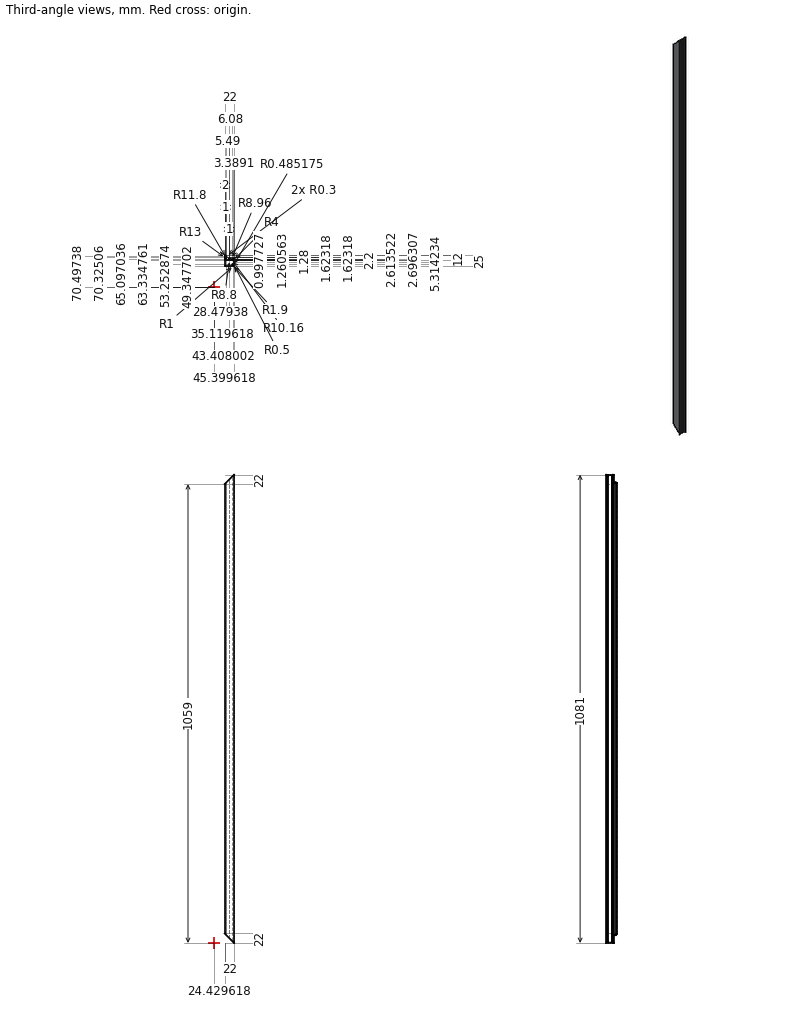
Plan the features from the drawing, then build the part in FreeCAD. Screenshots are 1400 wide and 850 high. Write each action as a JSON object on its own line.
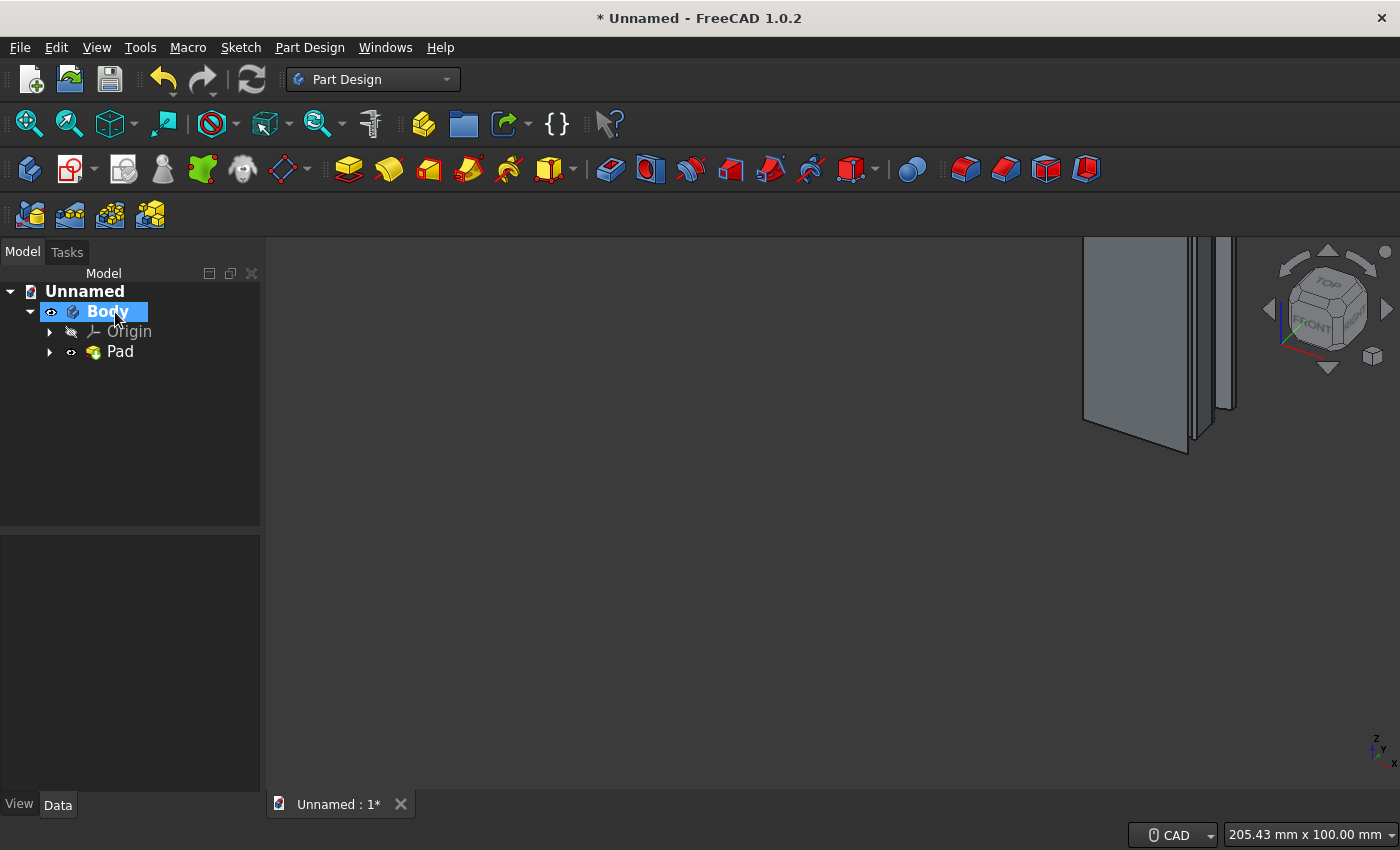
{"action": "left_click", "coordinate": [30, 124]}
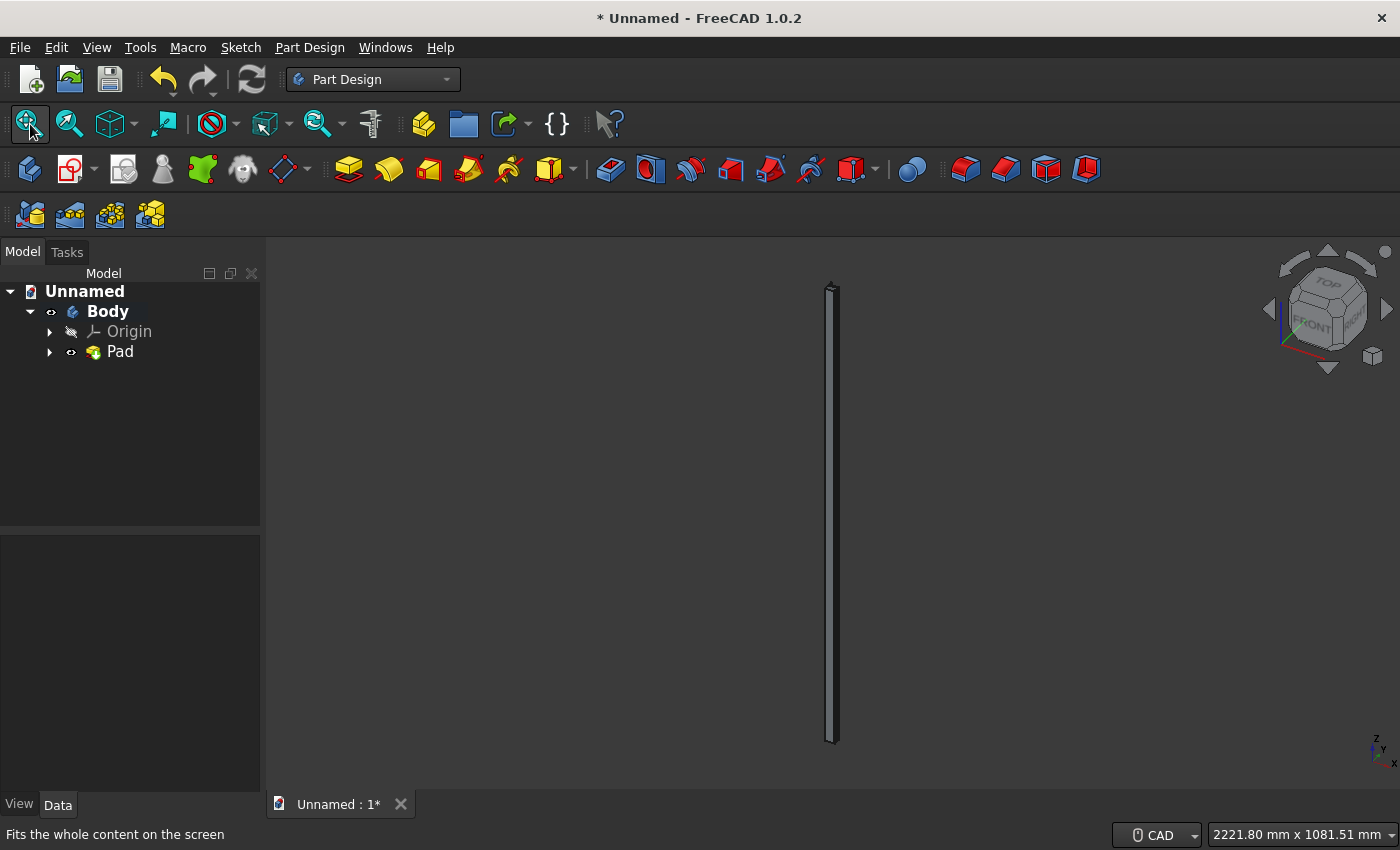
{"action": "scroll", "coordinate": [830, 321], "scroll_direction": "up", "scroll_amount": 4}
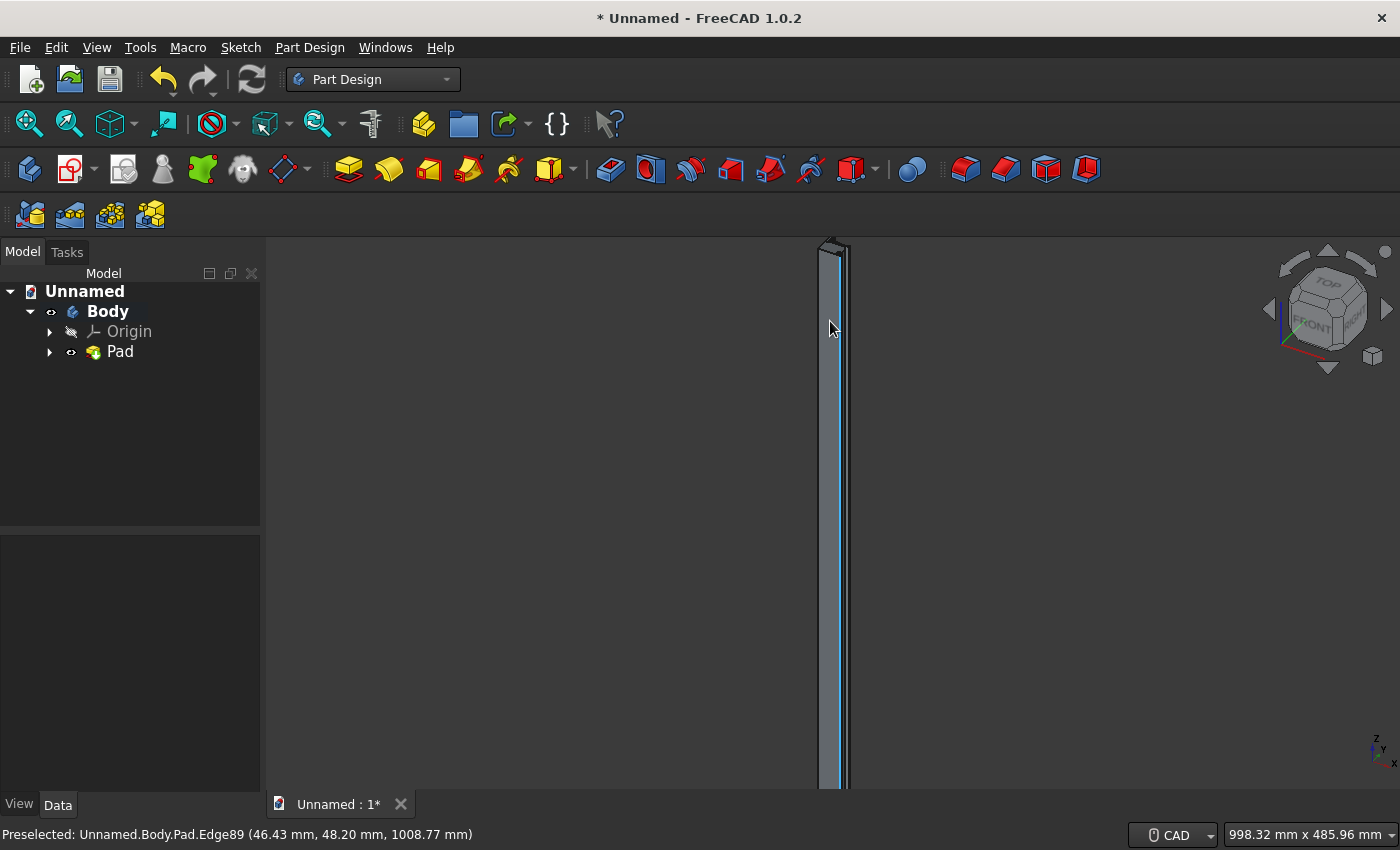
{"action": "left_click", "coordinate": [829, 323]}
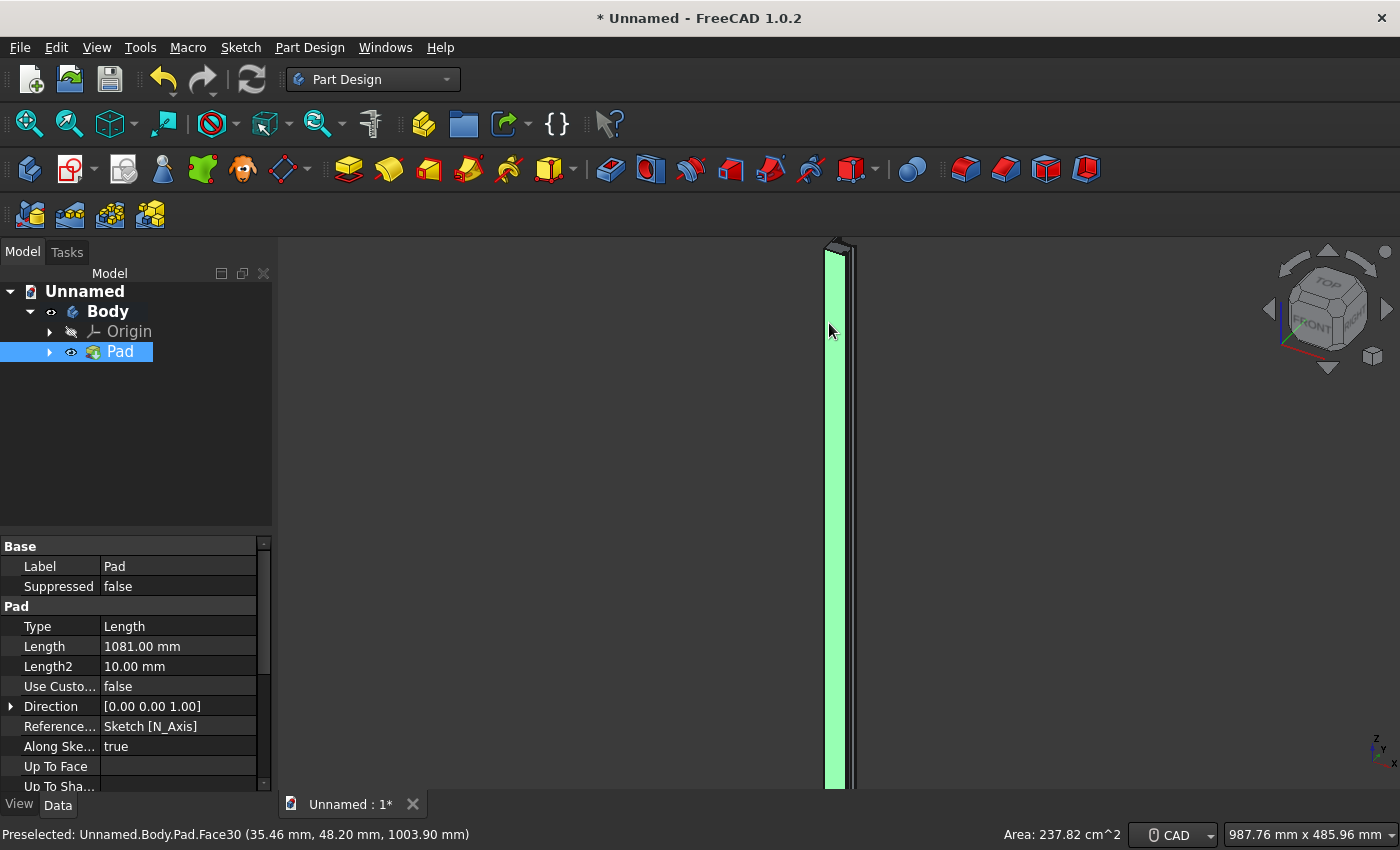
{"action": "left_click", "coordinate": [70, 170]}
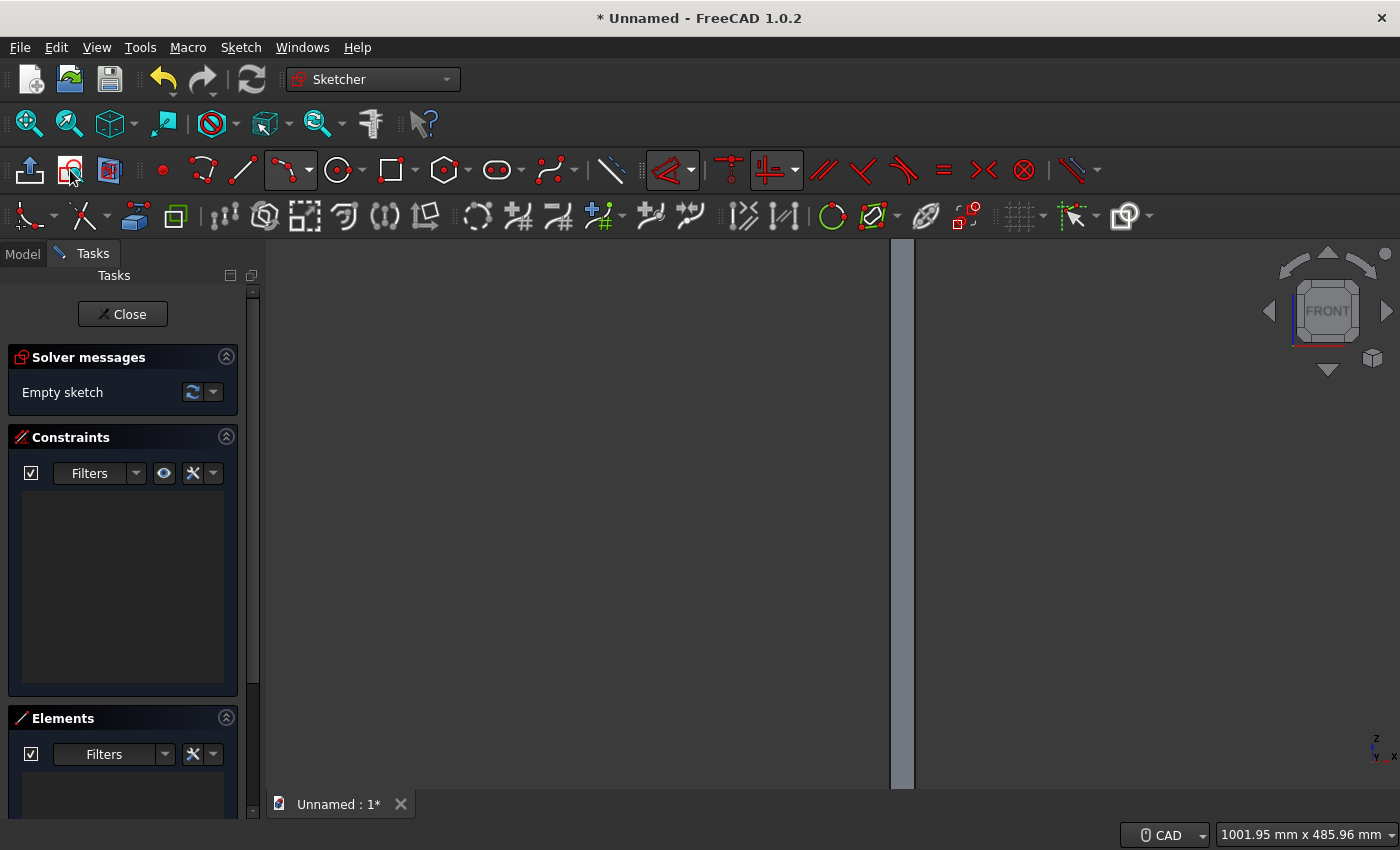
{"action": "scroll", "coordinate": [764, 514], "scroll_direction": "down", "scroll_amount": 5}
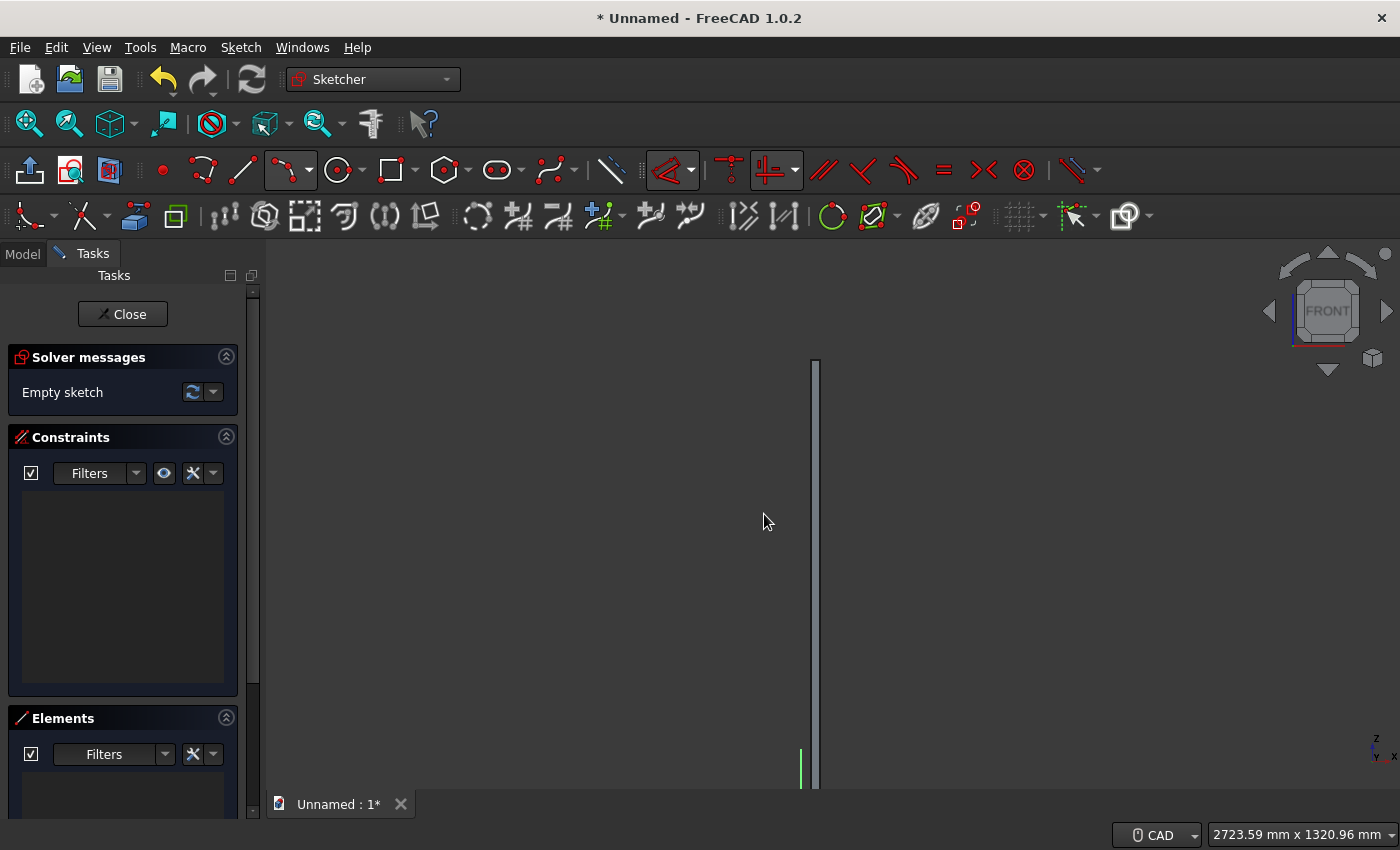
{"action": "scroll", "coordinate": [764, 514], "scroll_direction": "down", "scroll_amount": 5}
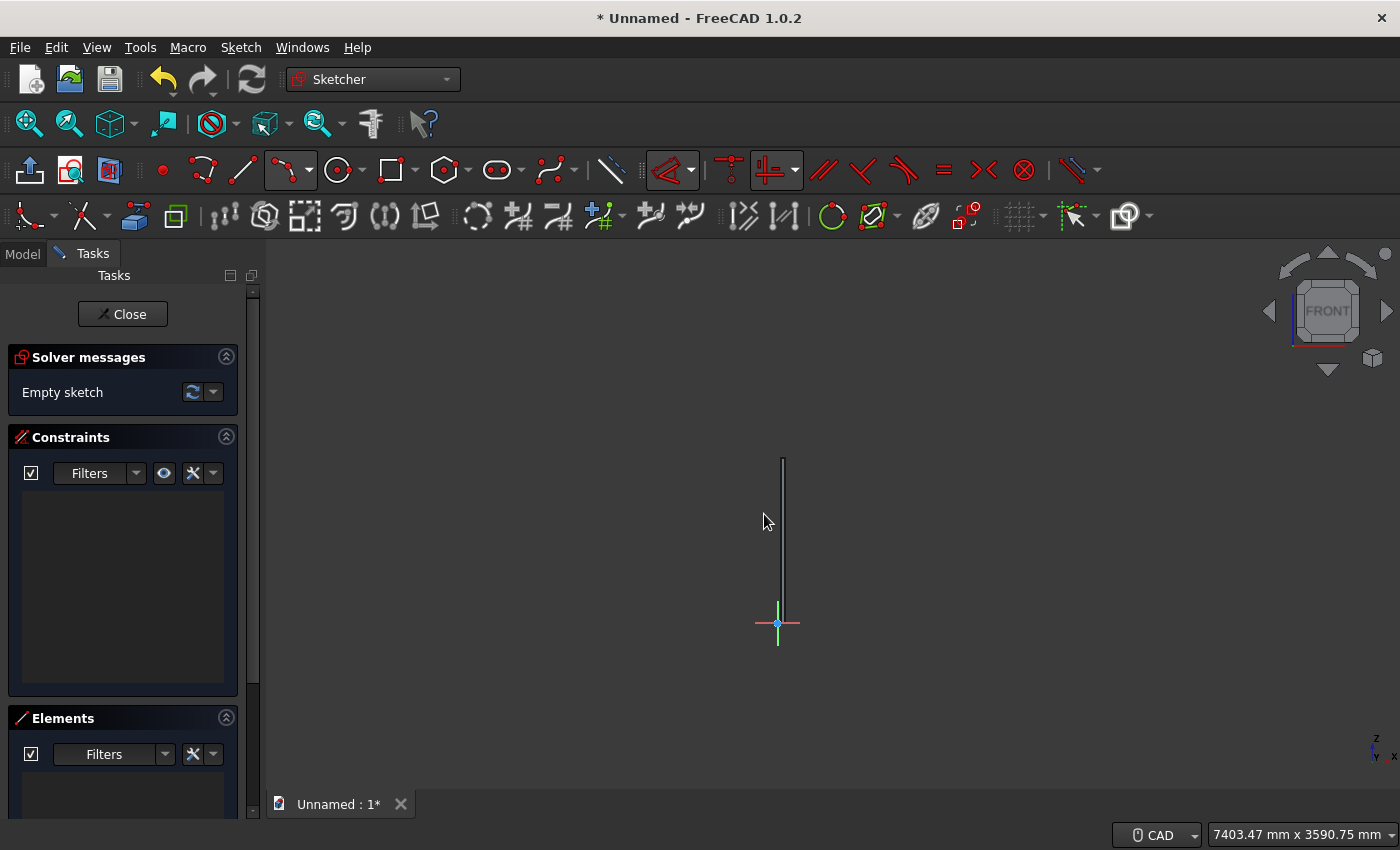
{"action": "scroll", "coordinate": [782, 627], "scroll_direction": "up", "scroll_amount": 15}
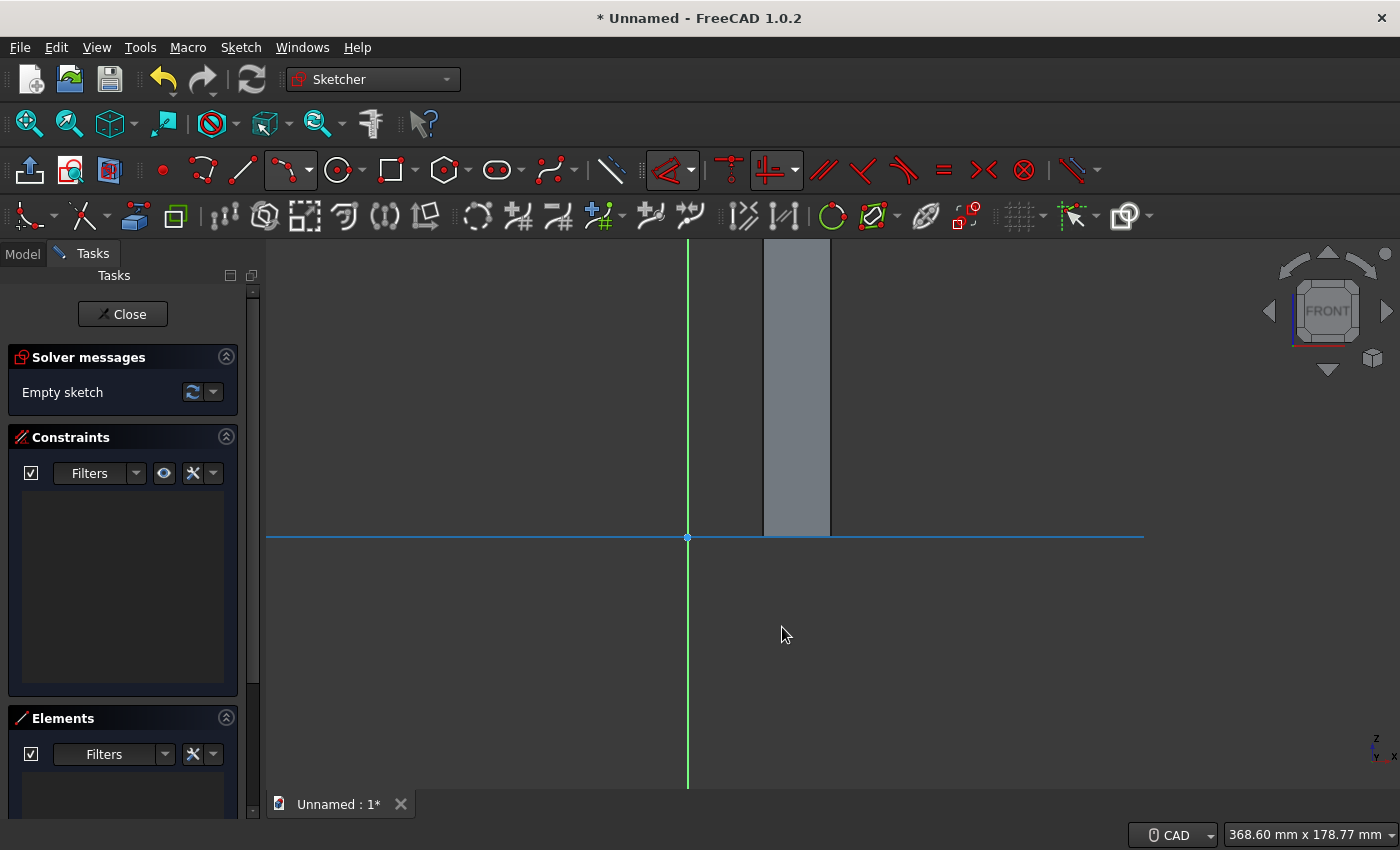
{"action": "scroll", "coordinate": [758, 500], "scroll_direction": "up", "scroll_amount": 8}